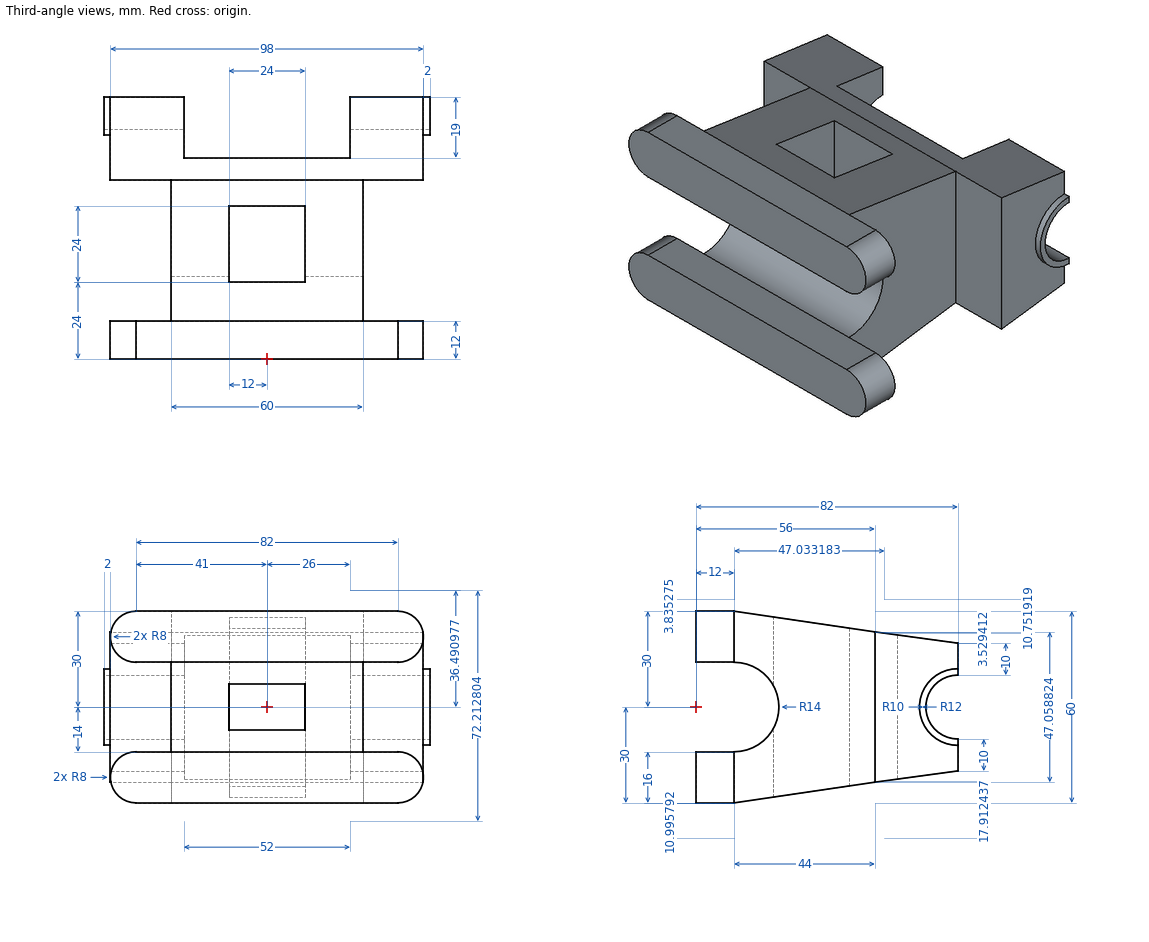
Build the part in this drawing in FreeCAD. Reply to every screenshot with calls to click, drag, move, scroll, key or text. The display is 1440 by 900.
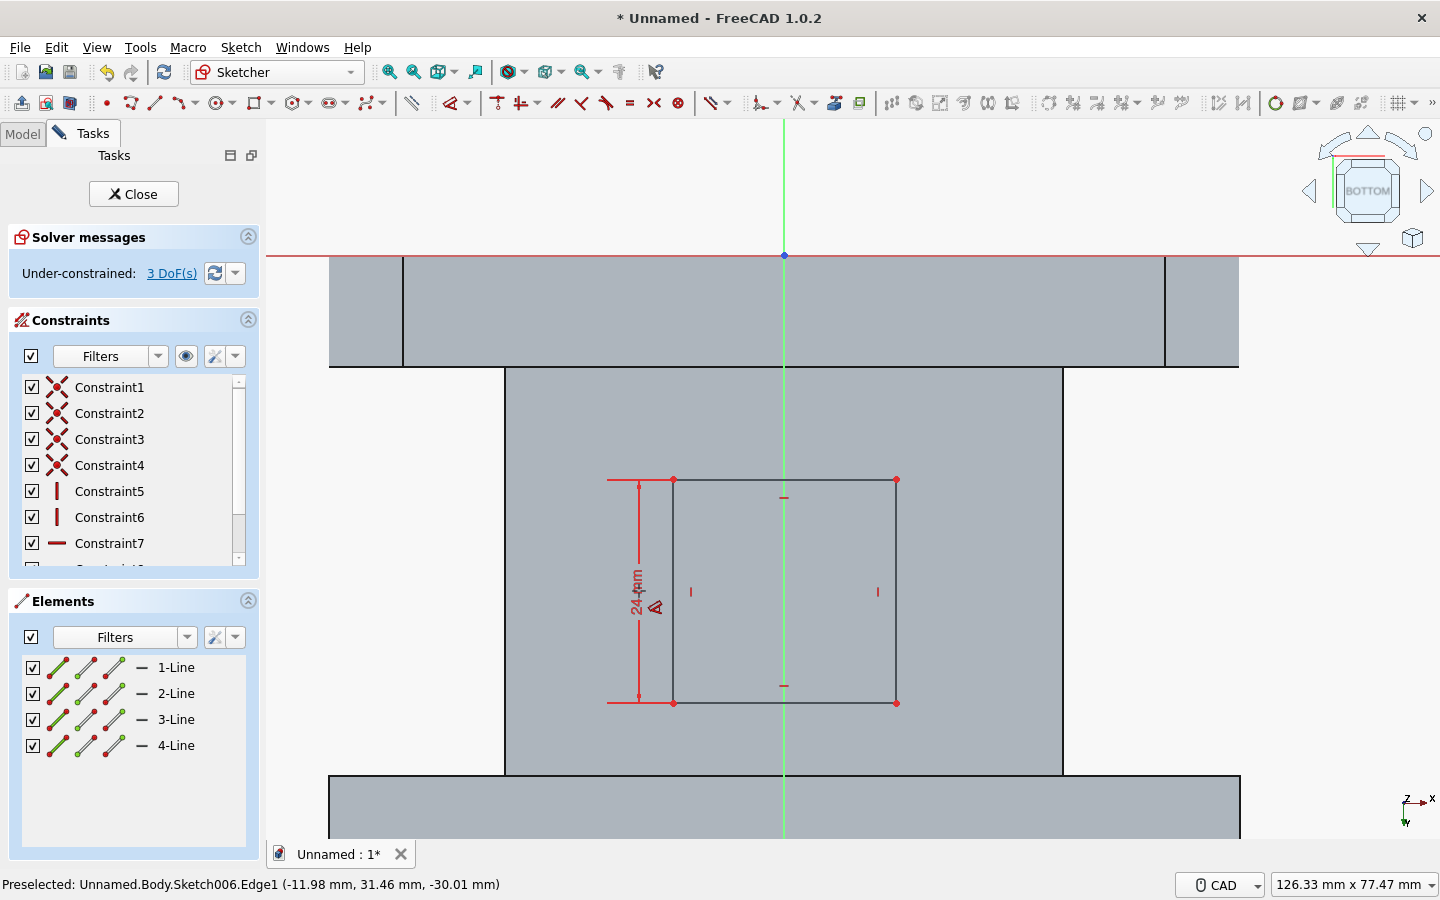
click(740, 703)
click(733, 737)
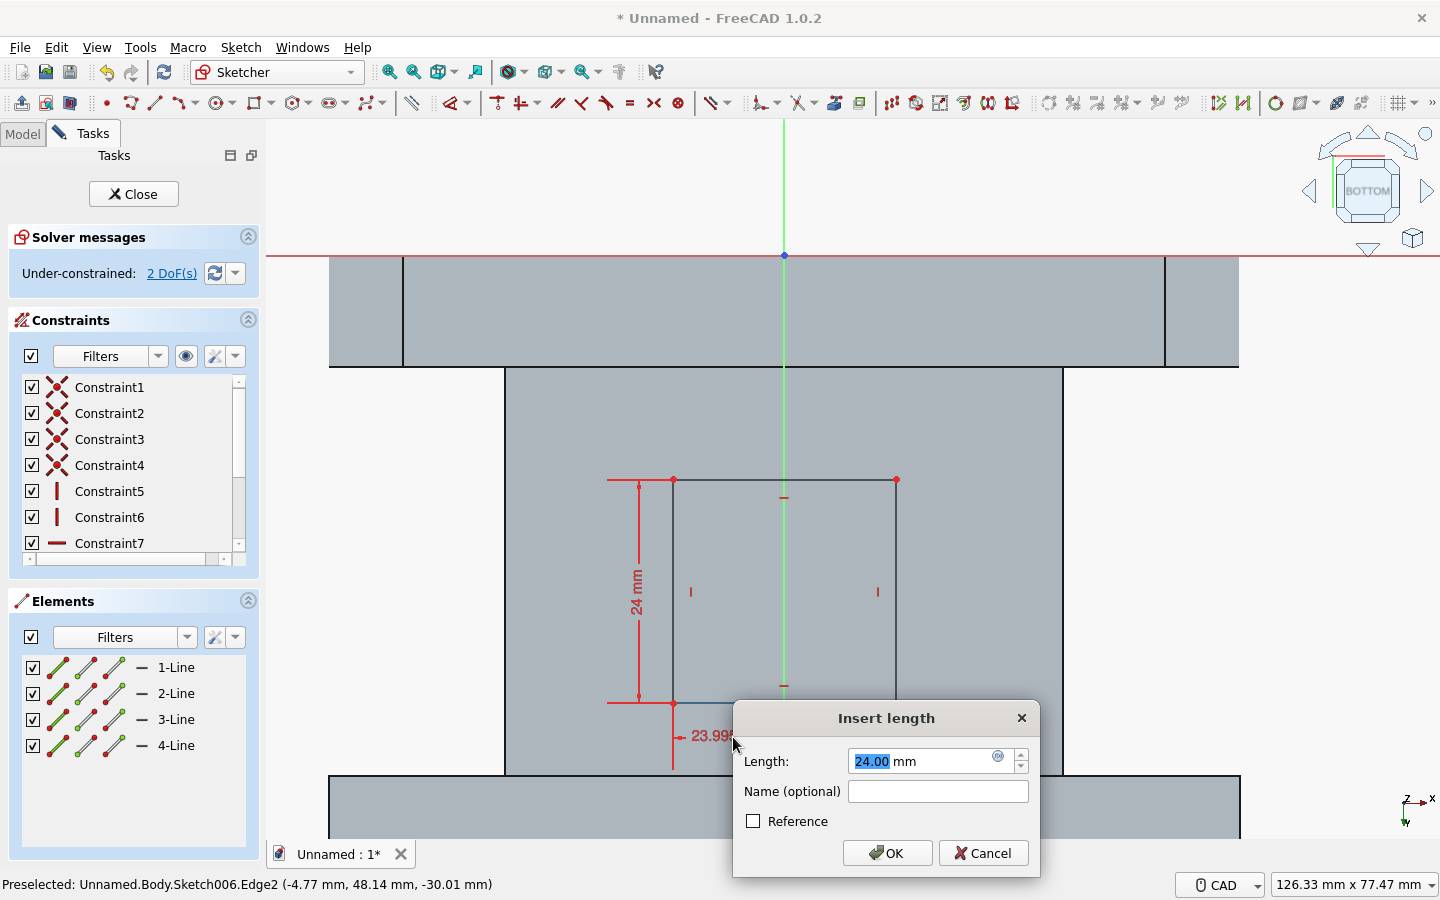
text(24)
key(Return)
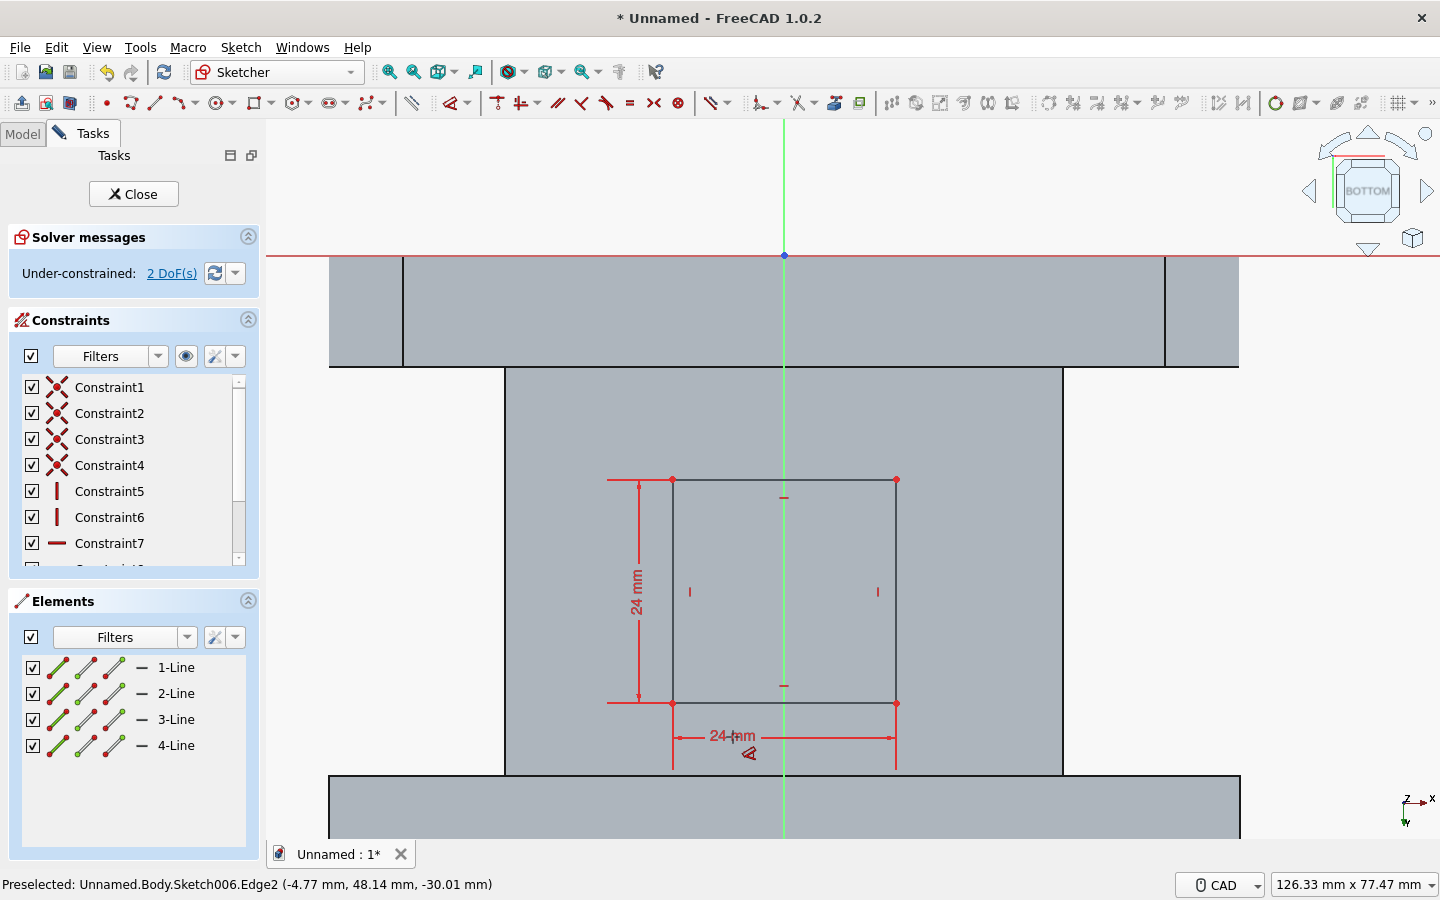
click(673, 480)
click(729, 222)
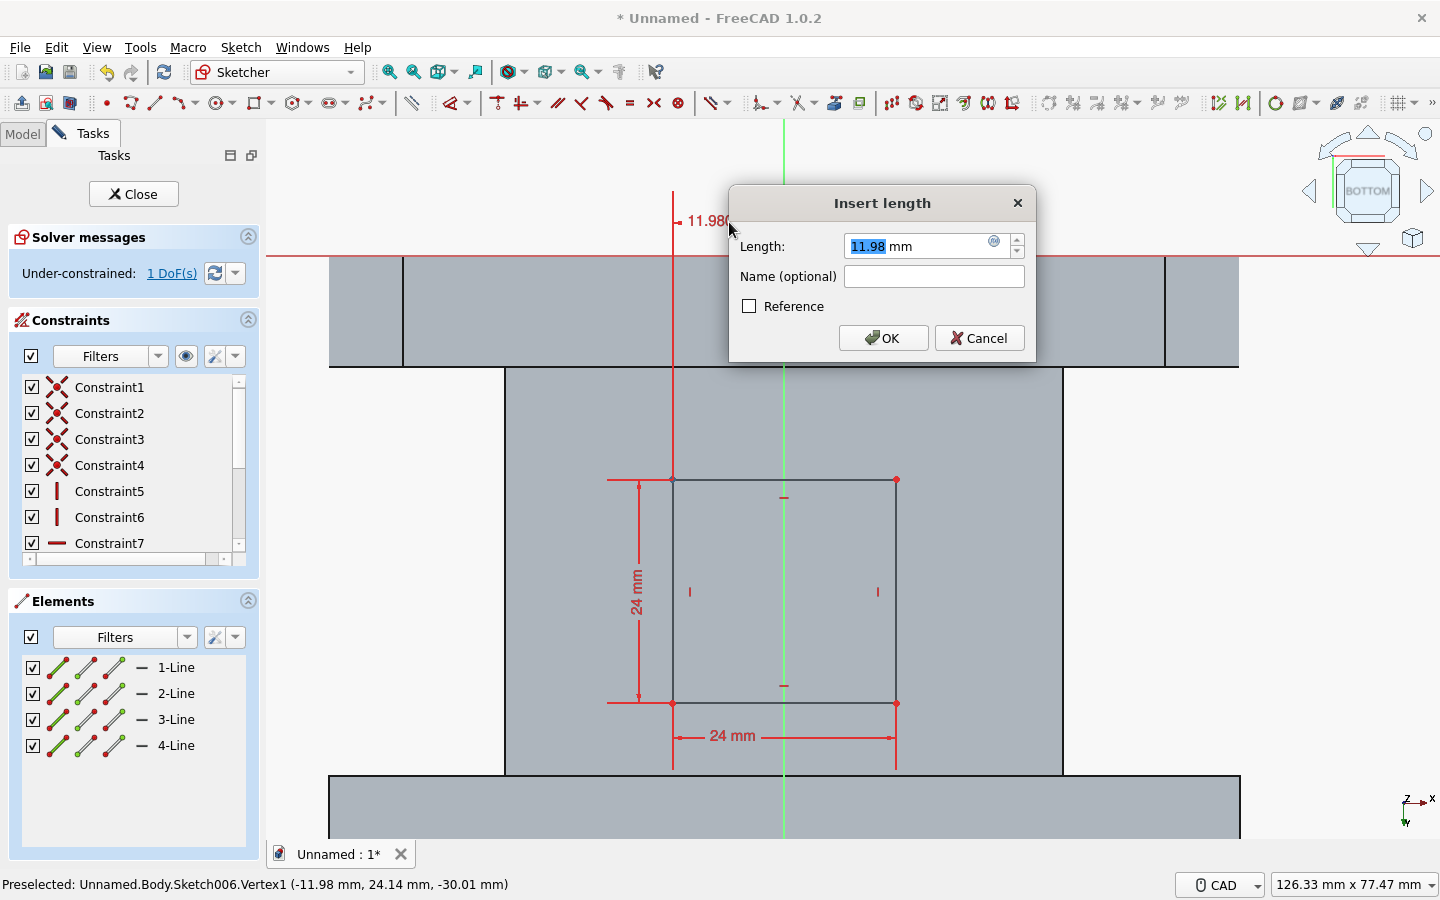
text(12)
key(Return)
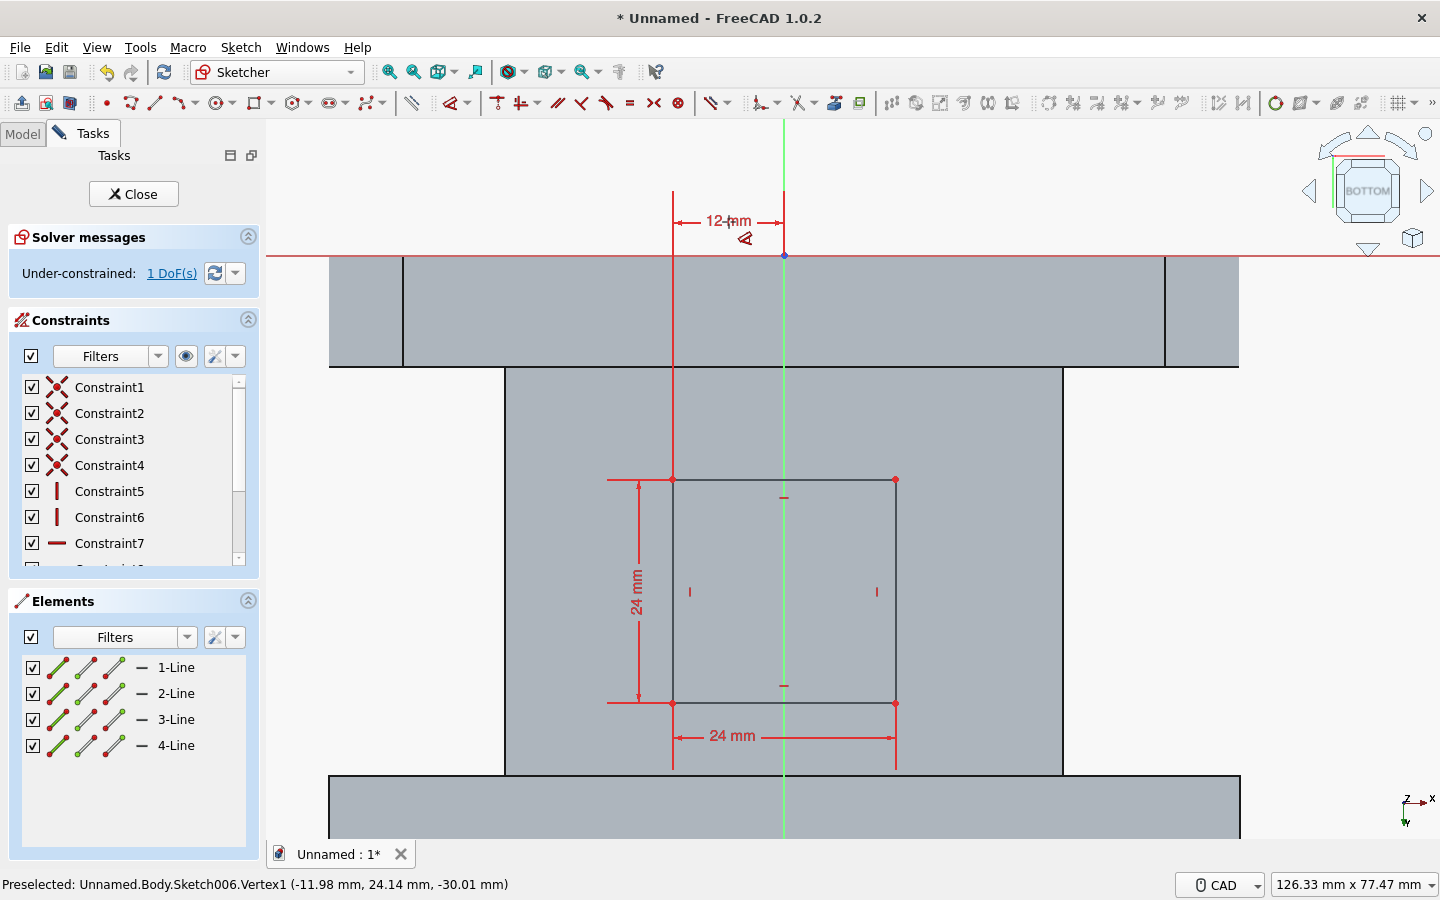
click(673, 480)
click(639, 368)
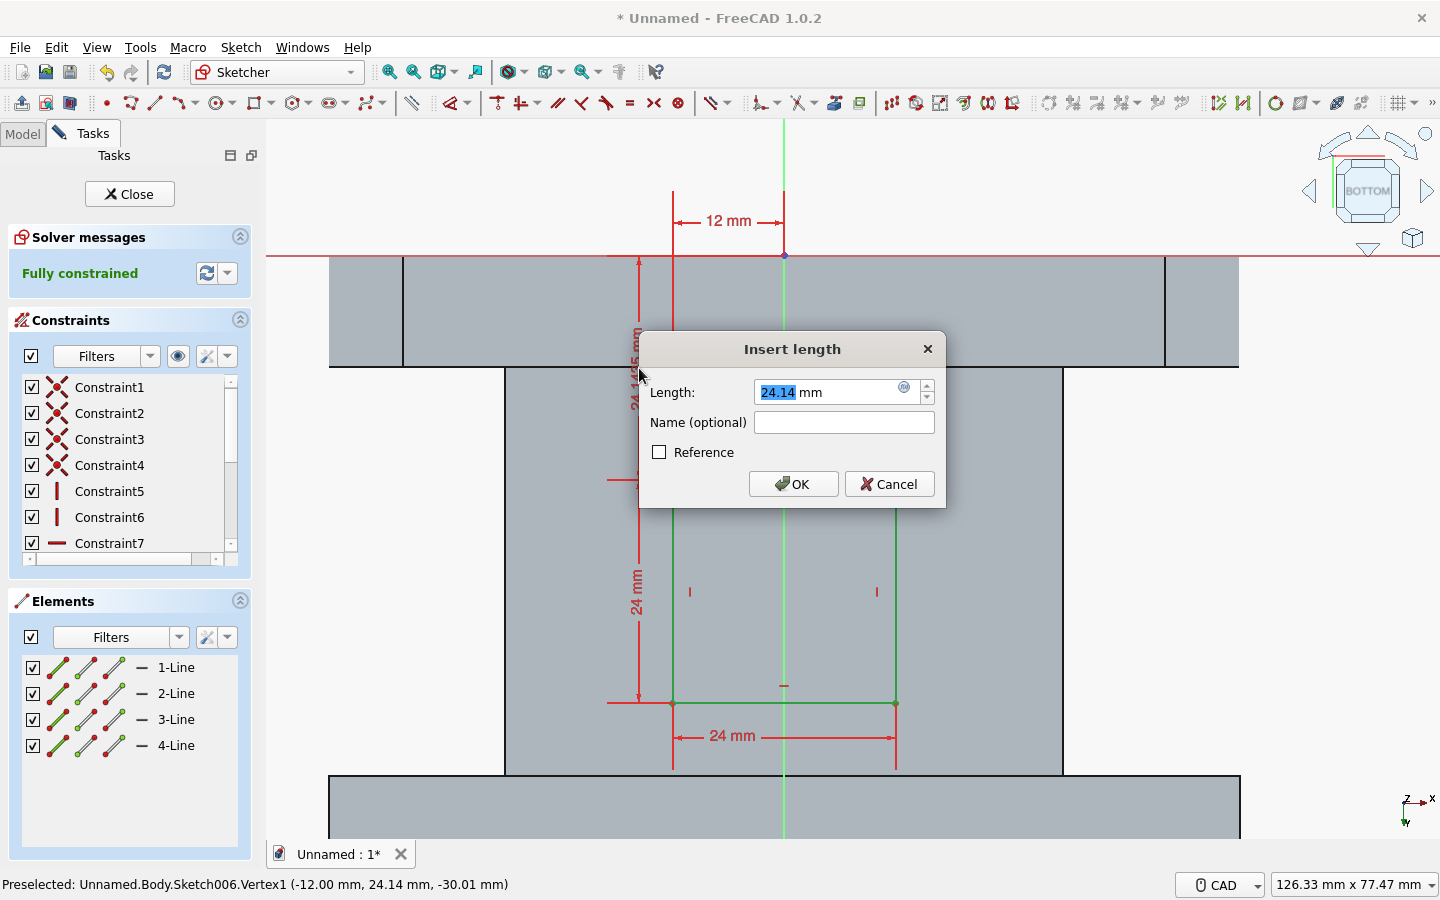
text(24)
key(Return)
key(Escape)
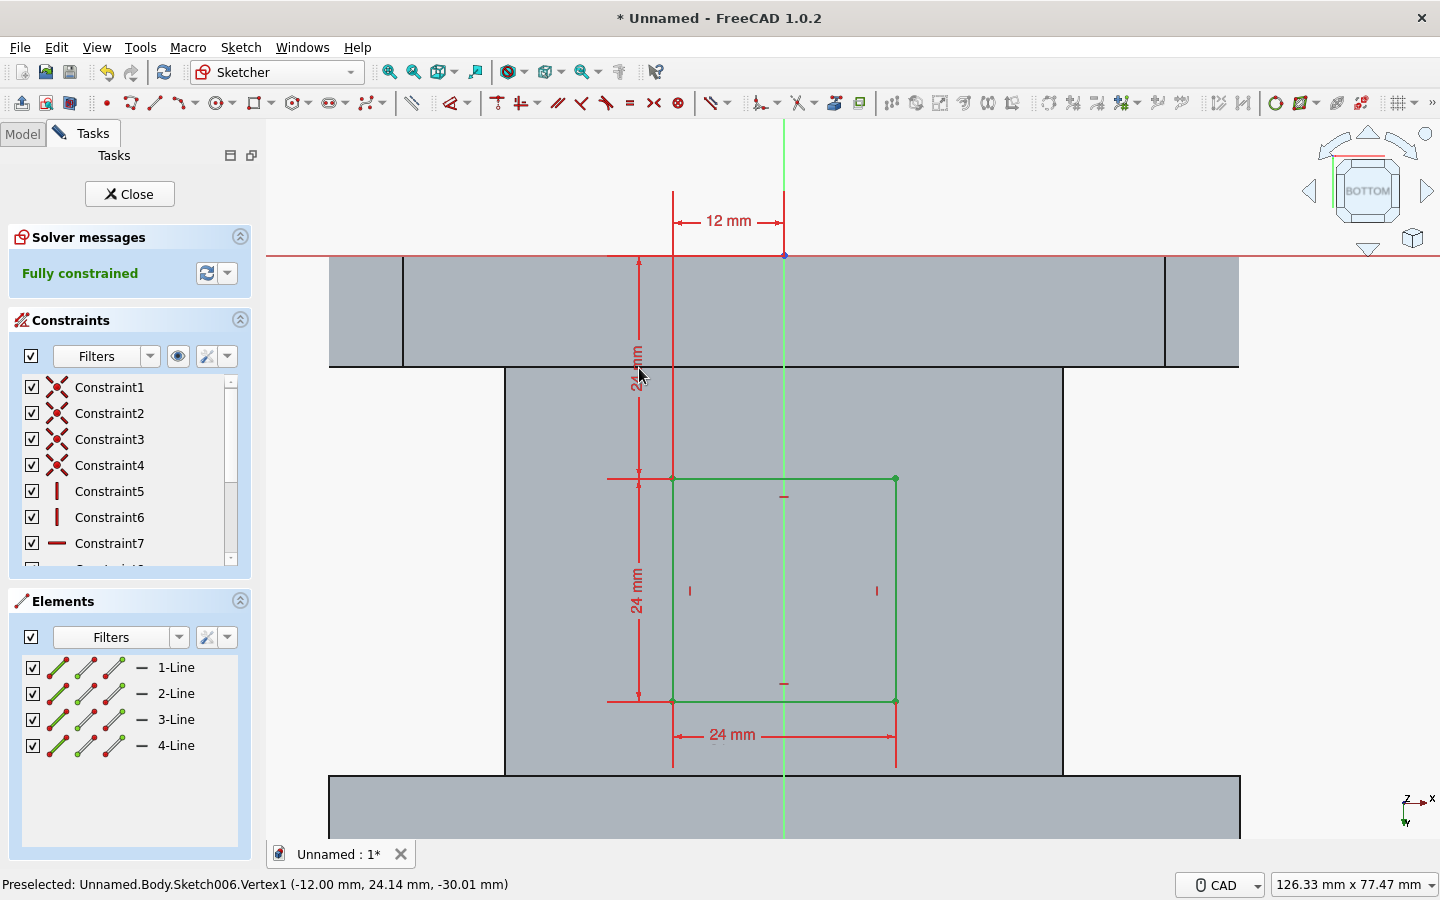
click(130, 194)